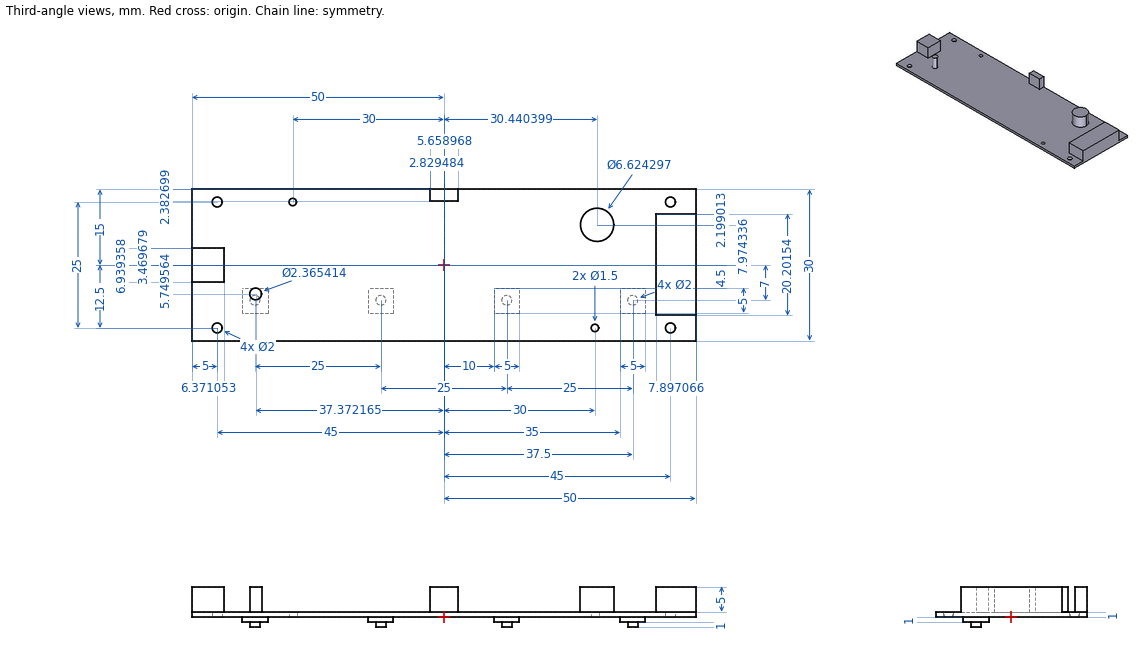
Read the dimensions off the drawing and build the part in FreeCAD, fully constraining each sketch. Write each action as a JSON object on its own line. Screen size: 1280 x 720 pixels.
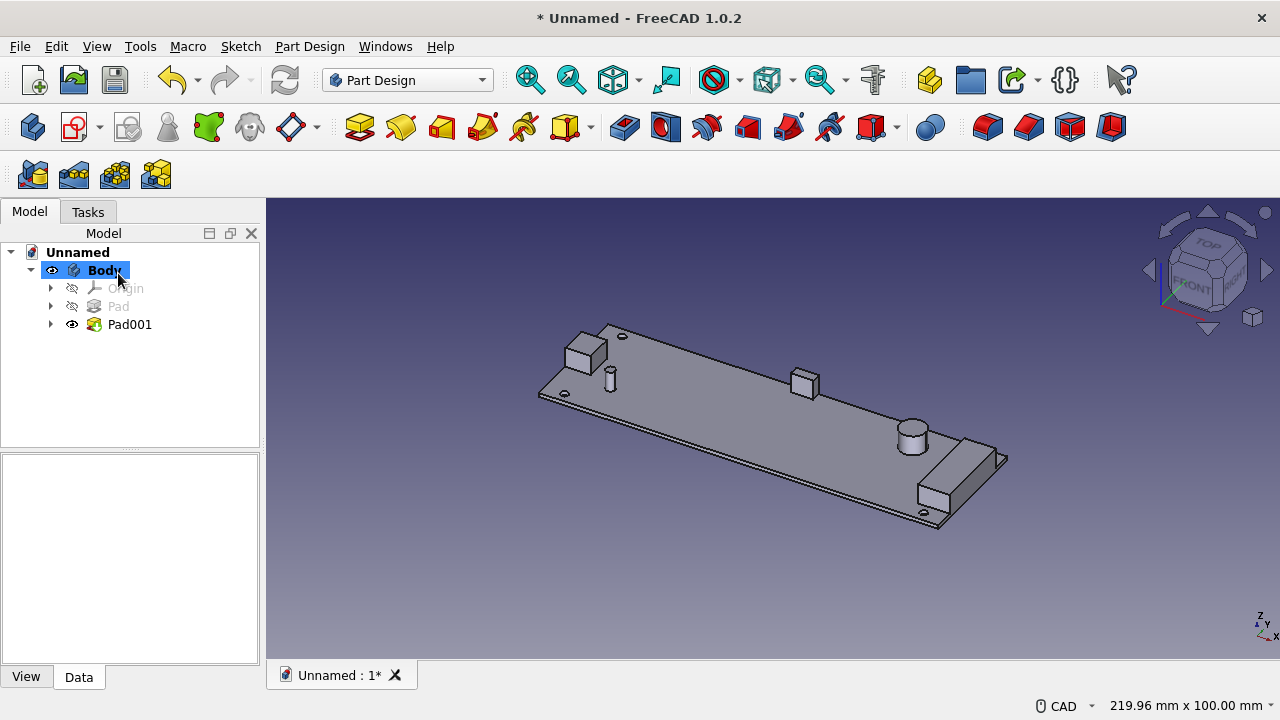
{"action": "left_click", "coordinate": [74, 128]}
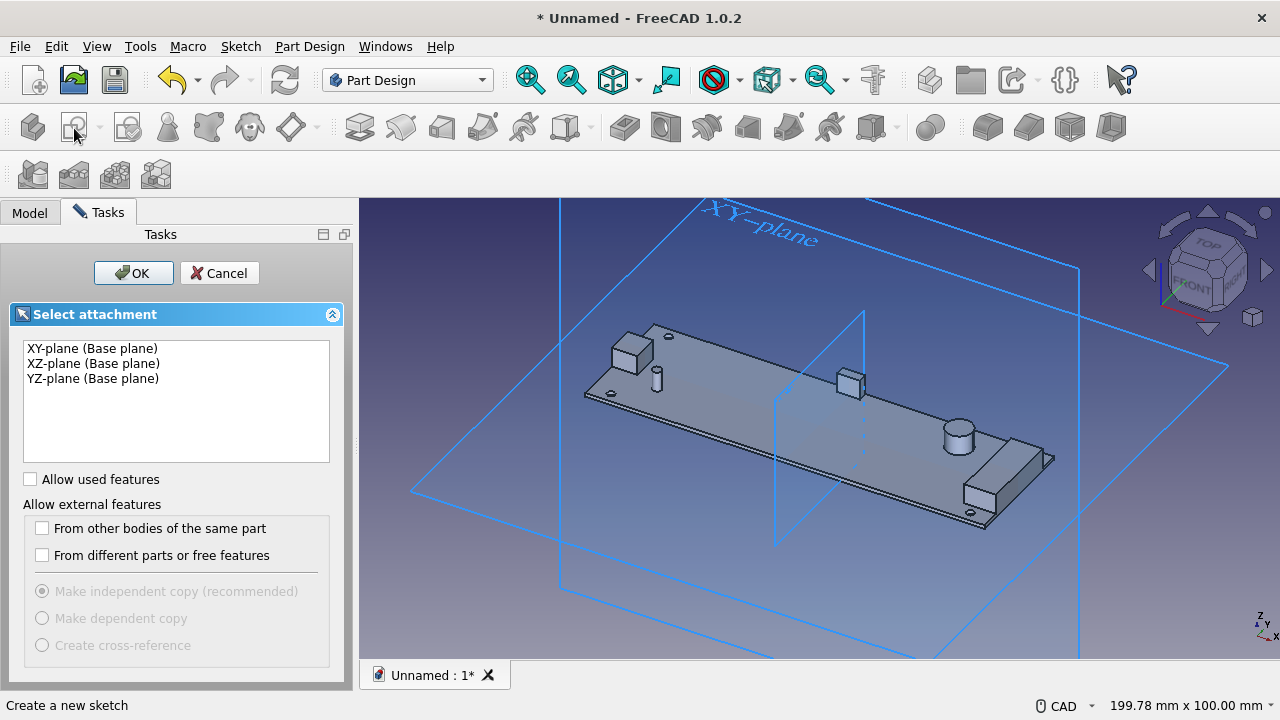
{"action": "left_click", "coordinate": [84, 348]}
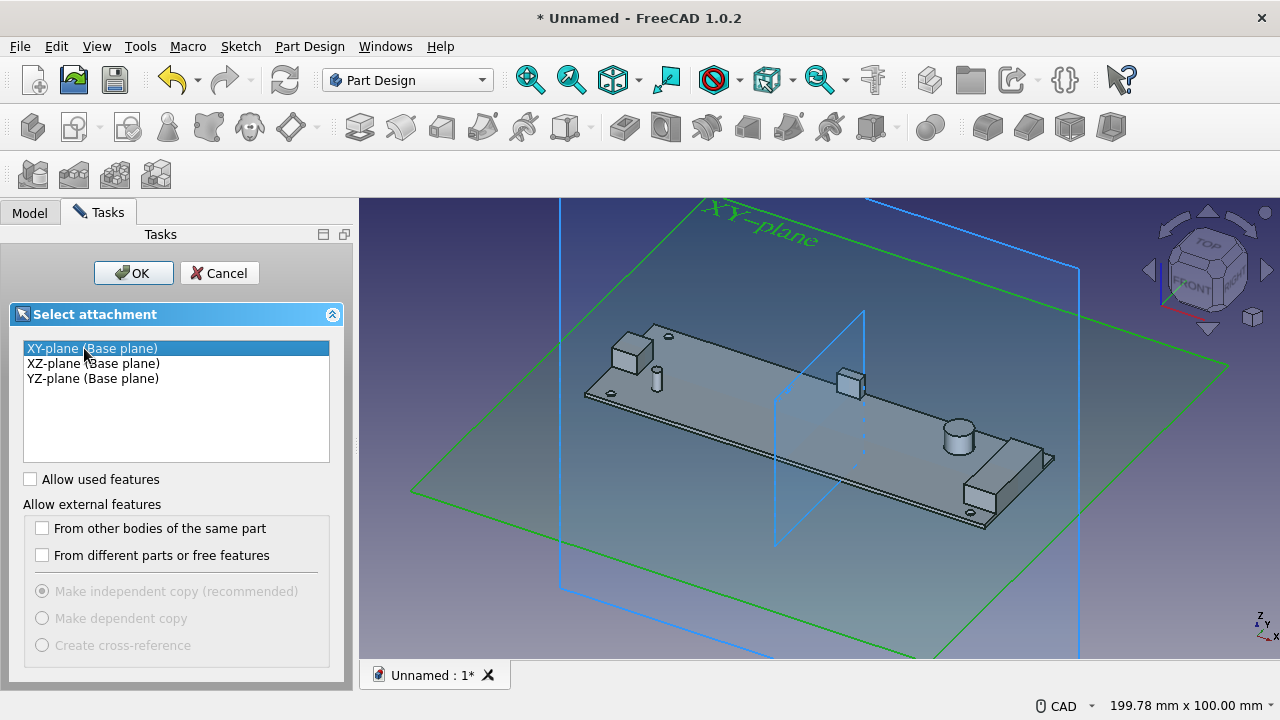
{"action": "left_click", "coordinate": [134, 273]}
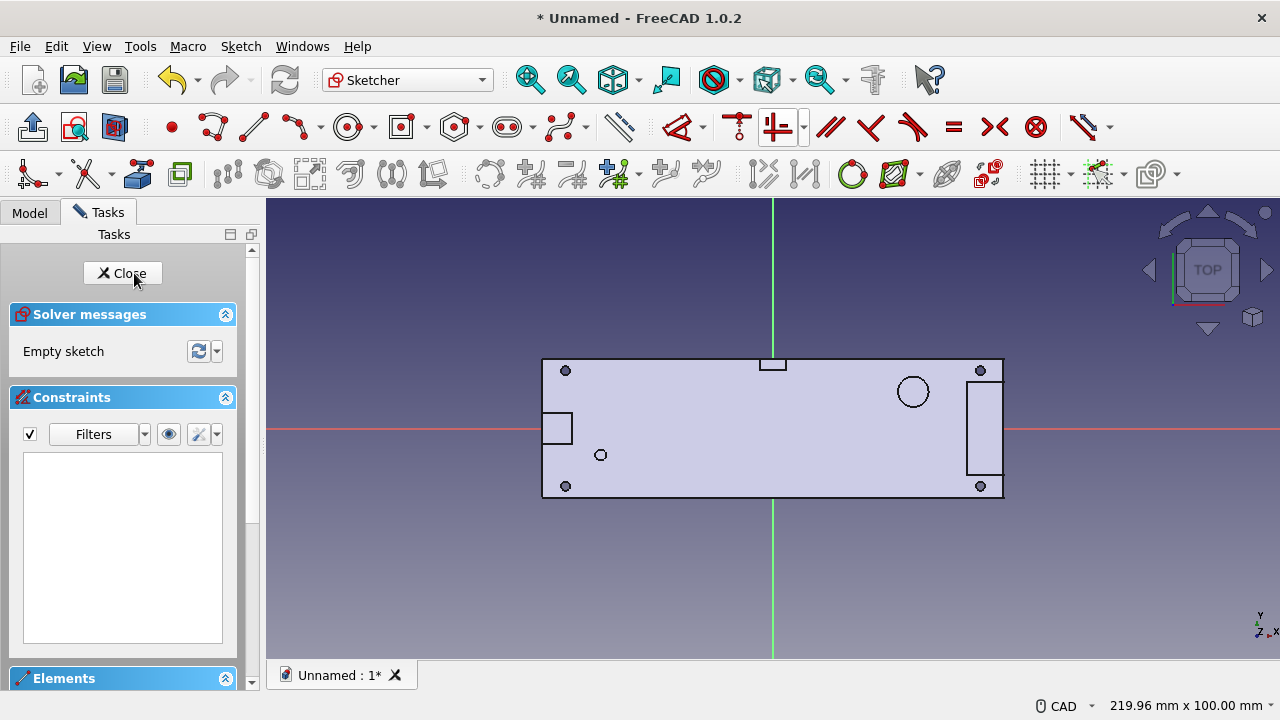
{"action": "left_click", "coordinate": [115, 128]}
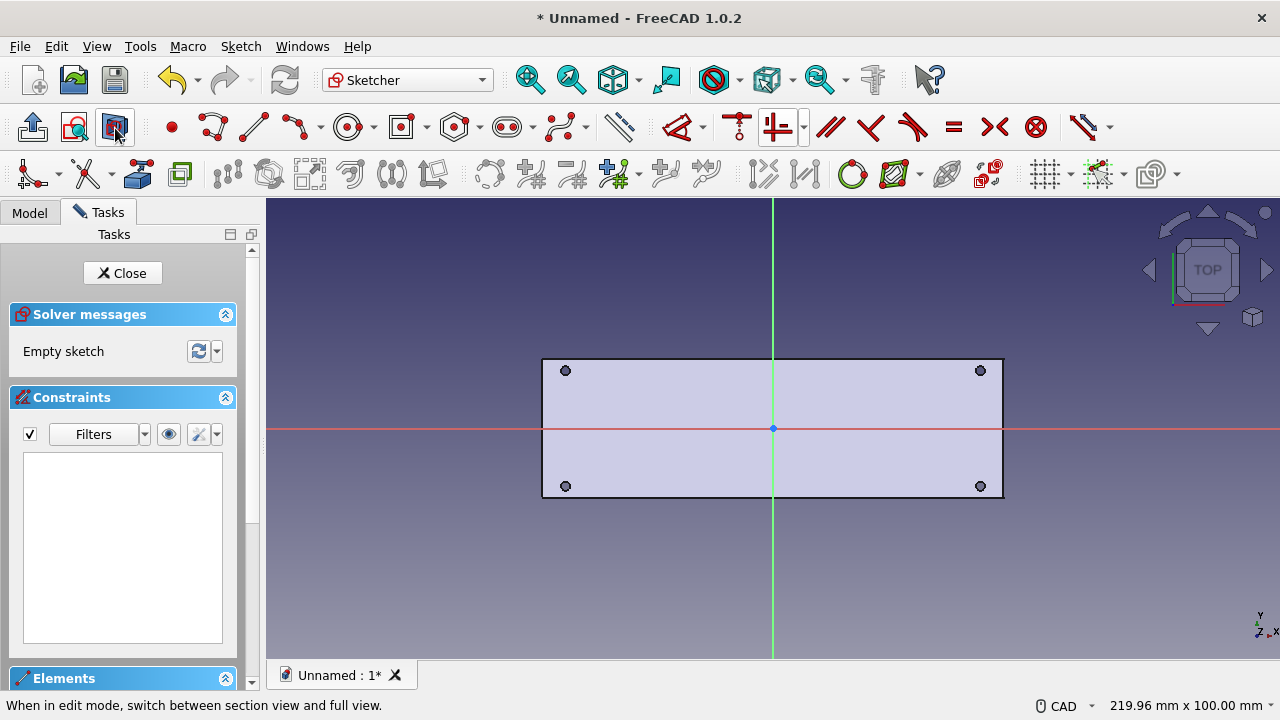
{"action": "scroll", "coordinate": [912, 495], "scroll_direction": "up", "scroll_amount": 2}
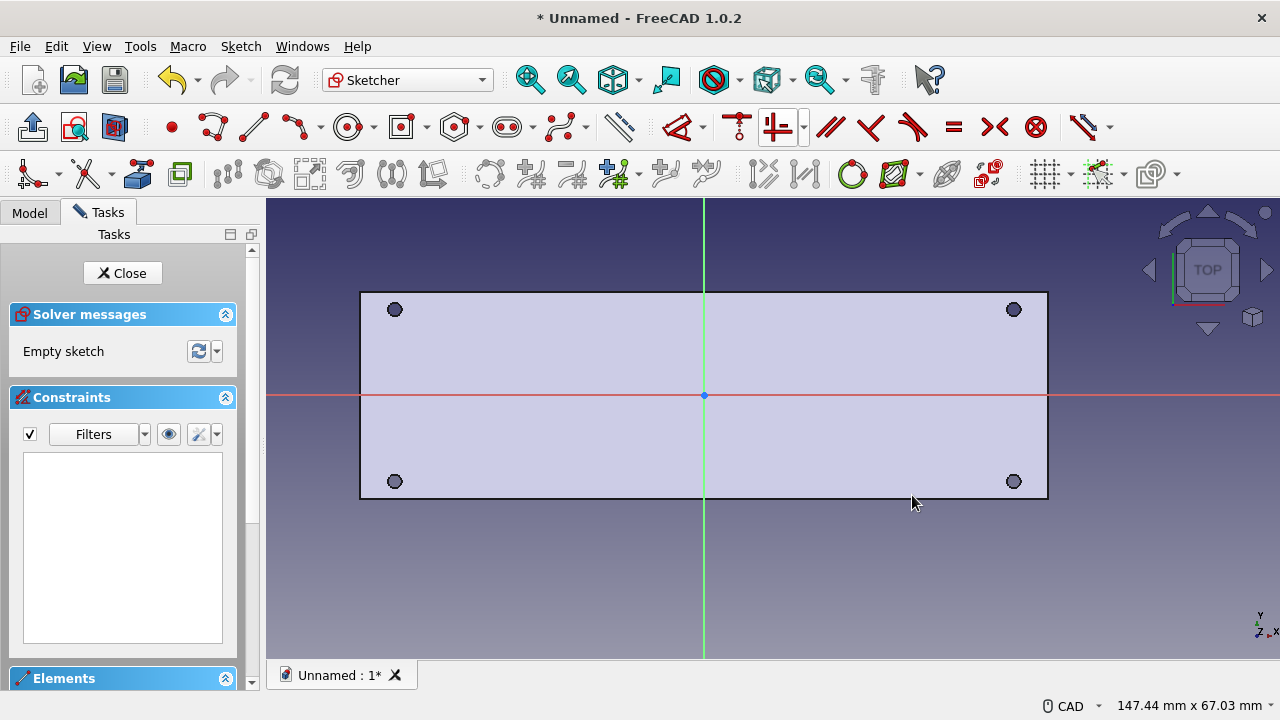
{"action": "left_click", "coordinate": [426, 128]}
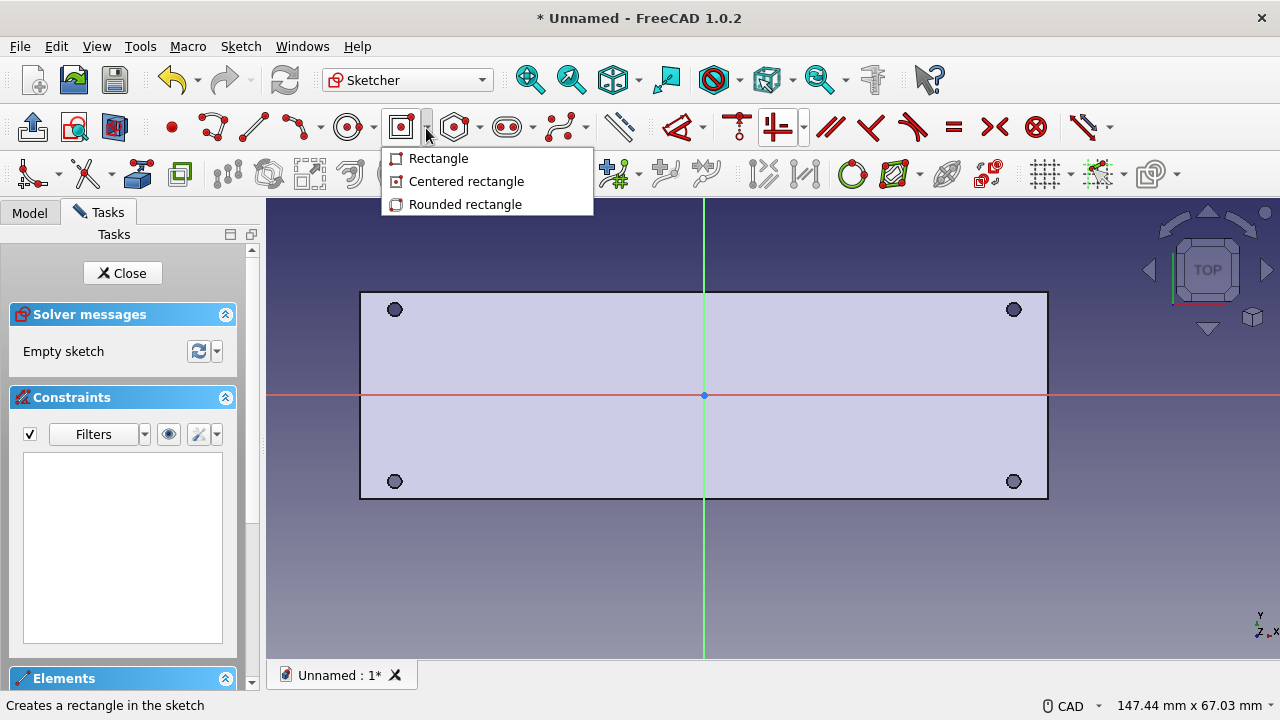
{"action": "left_click", "coordinate": [488, 158]}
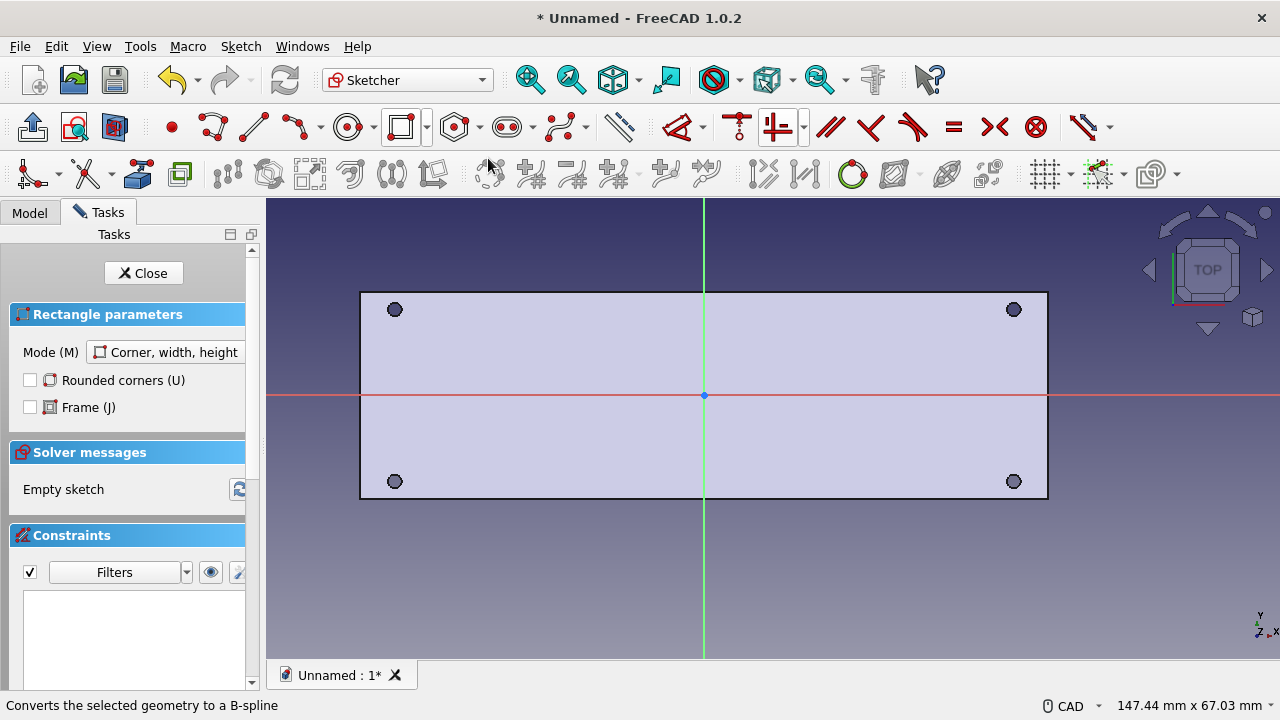
{"action": "left_click", "coordinate": [773, 426]}
{"action": "left_click", "coordinate": [807, 461]}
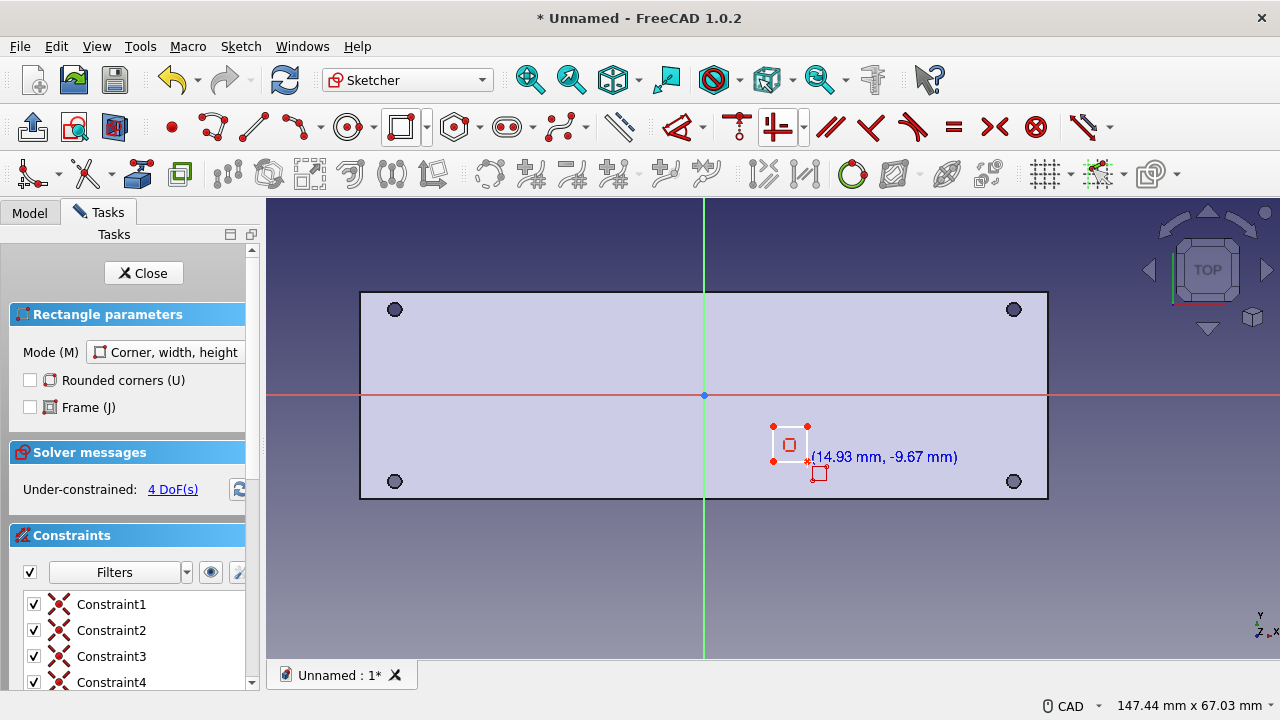
{"action": "left_click", "coordinate": [945, 426]}
{"action": "left_click", "coordinate": [979, 461]}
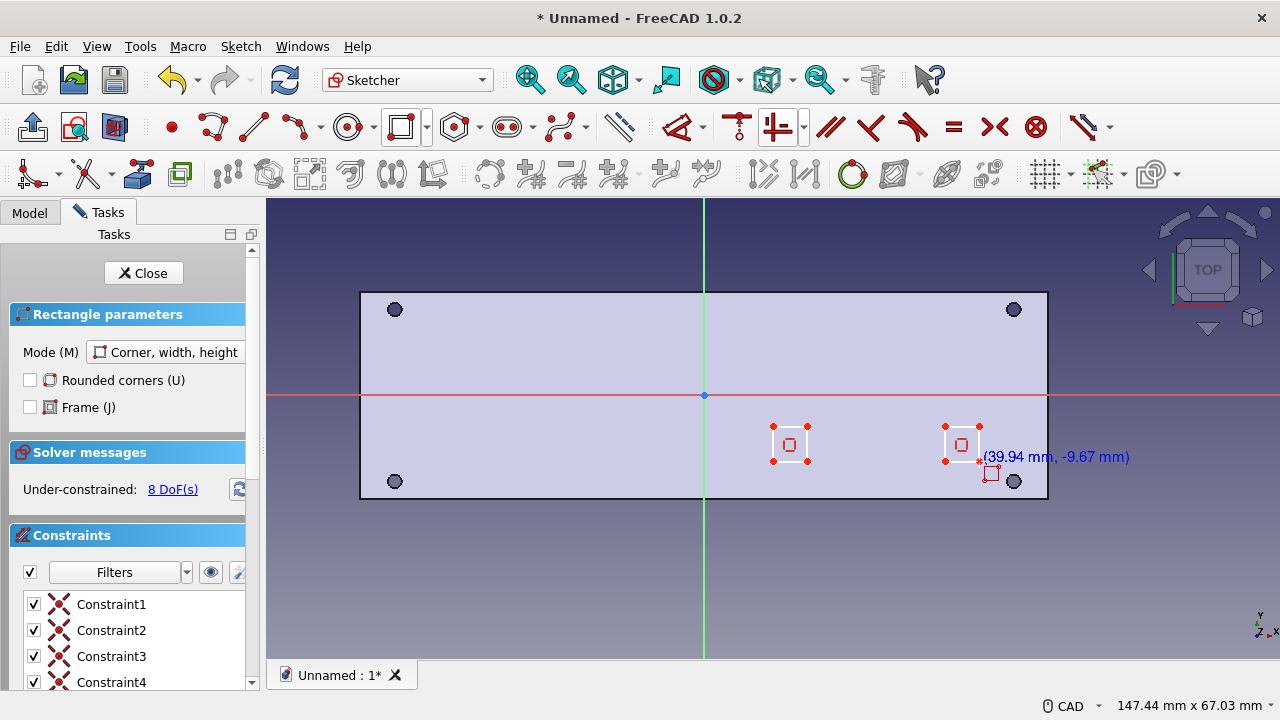
{"action": "left_click", "coordinate": [429, 426]}
{"action": "left_click", "coordinate": [464, 461]}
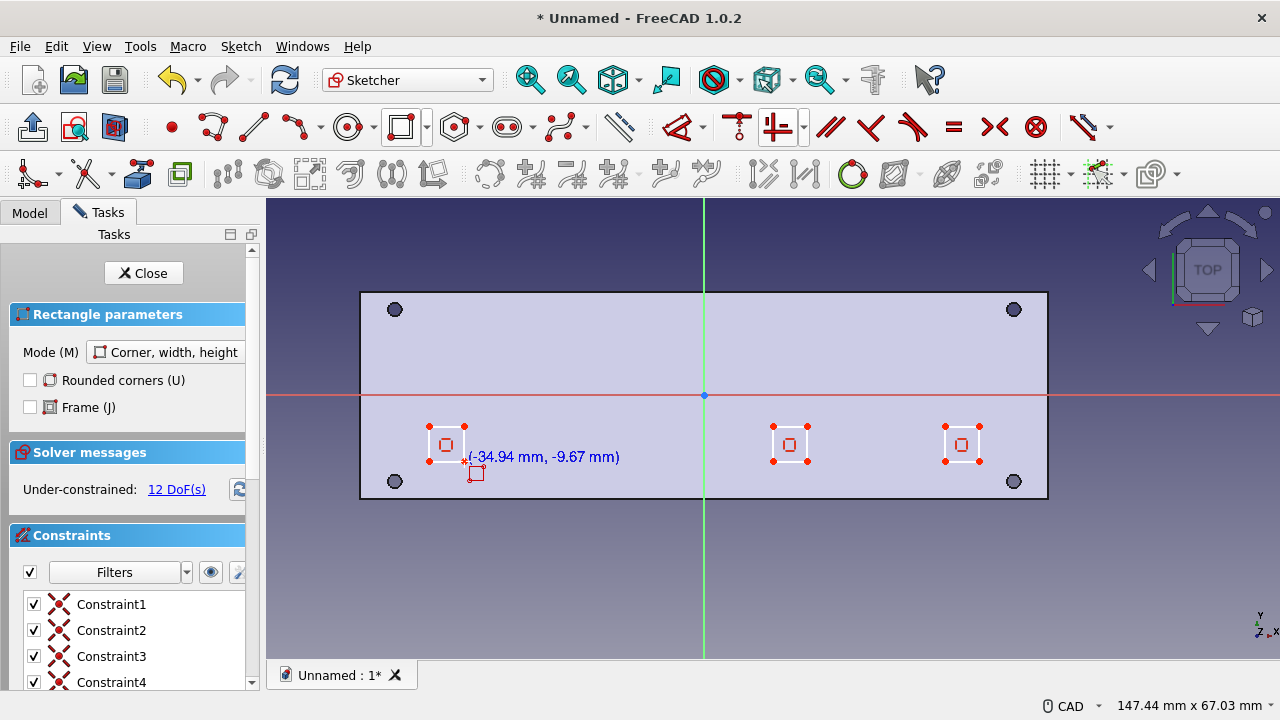
{"action": "left_click", "coordinate": [601, 426]}
{"action": "left_click", "coordinate": [636, 461]}
{"action": "key", "text": "Escape"}